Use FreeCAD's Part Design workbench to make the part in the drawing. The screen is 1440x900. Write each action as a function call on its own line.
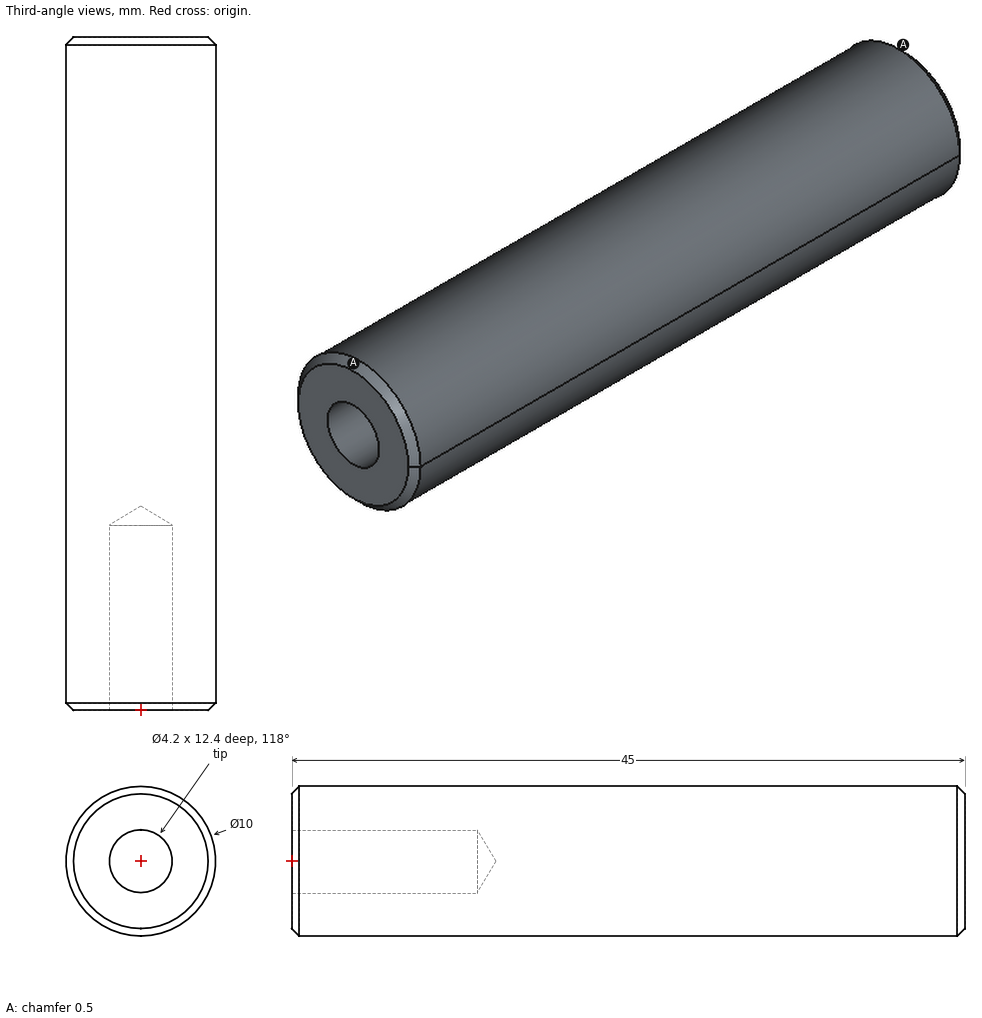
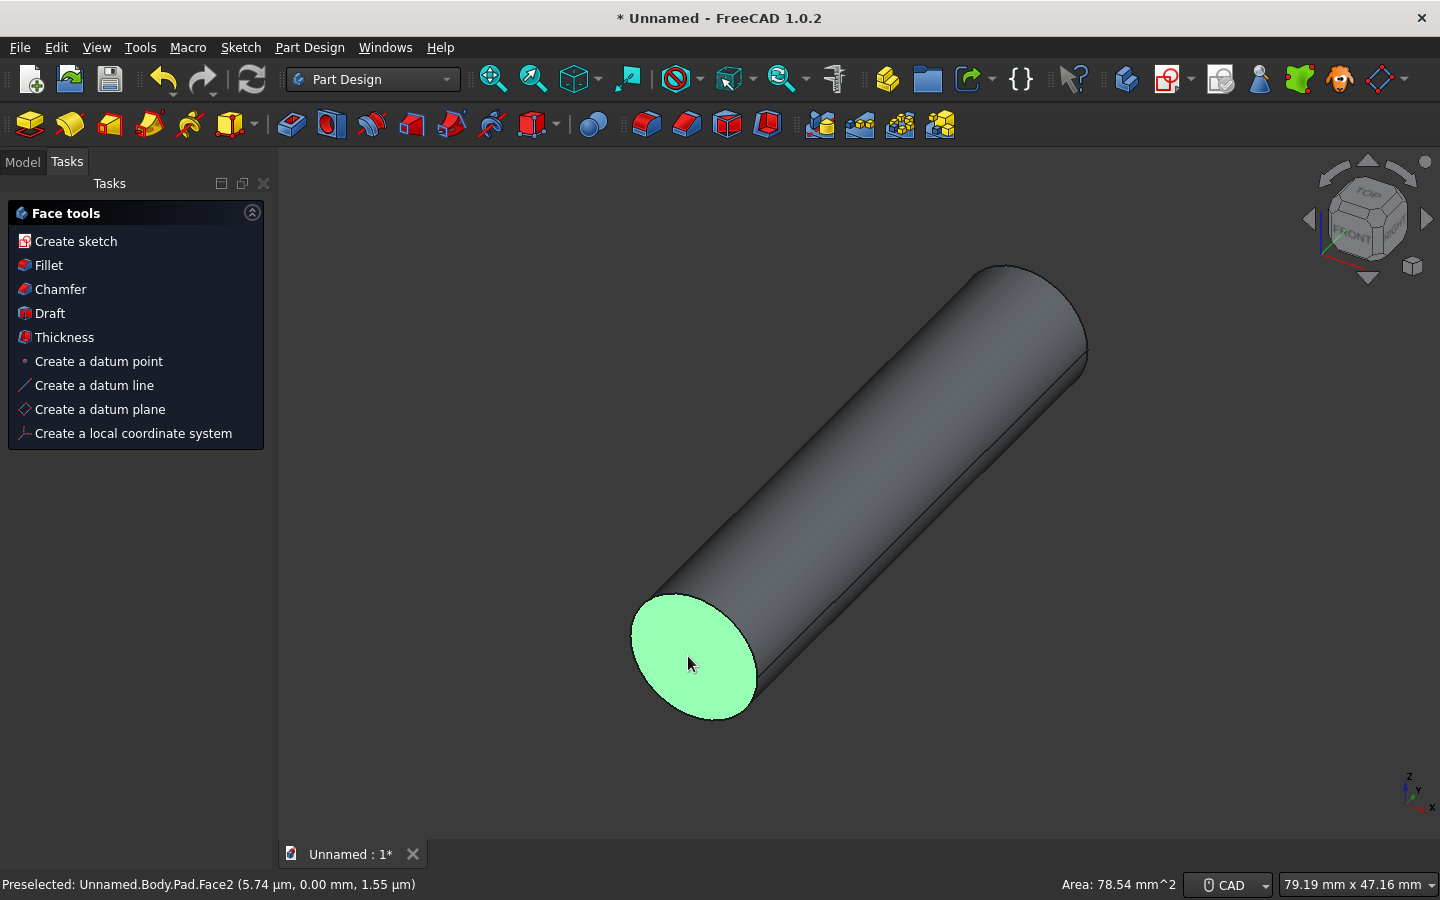
click(1168, 80)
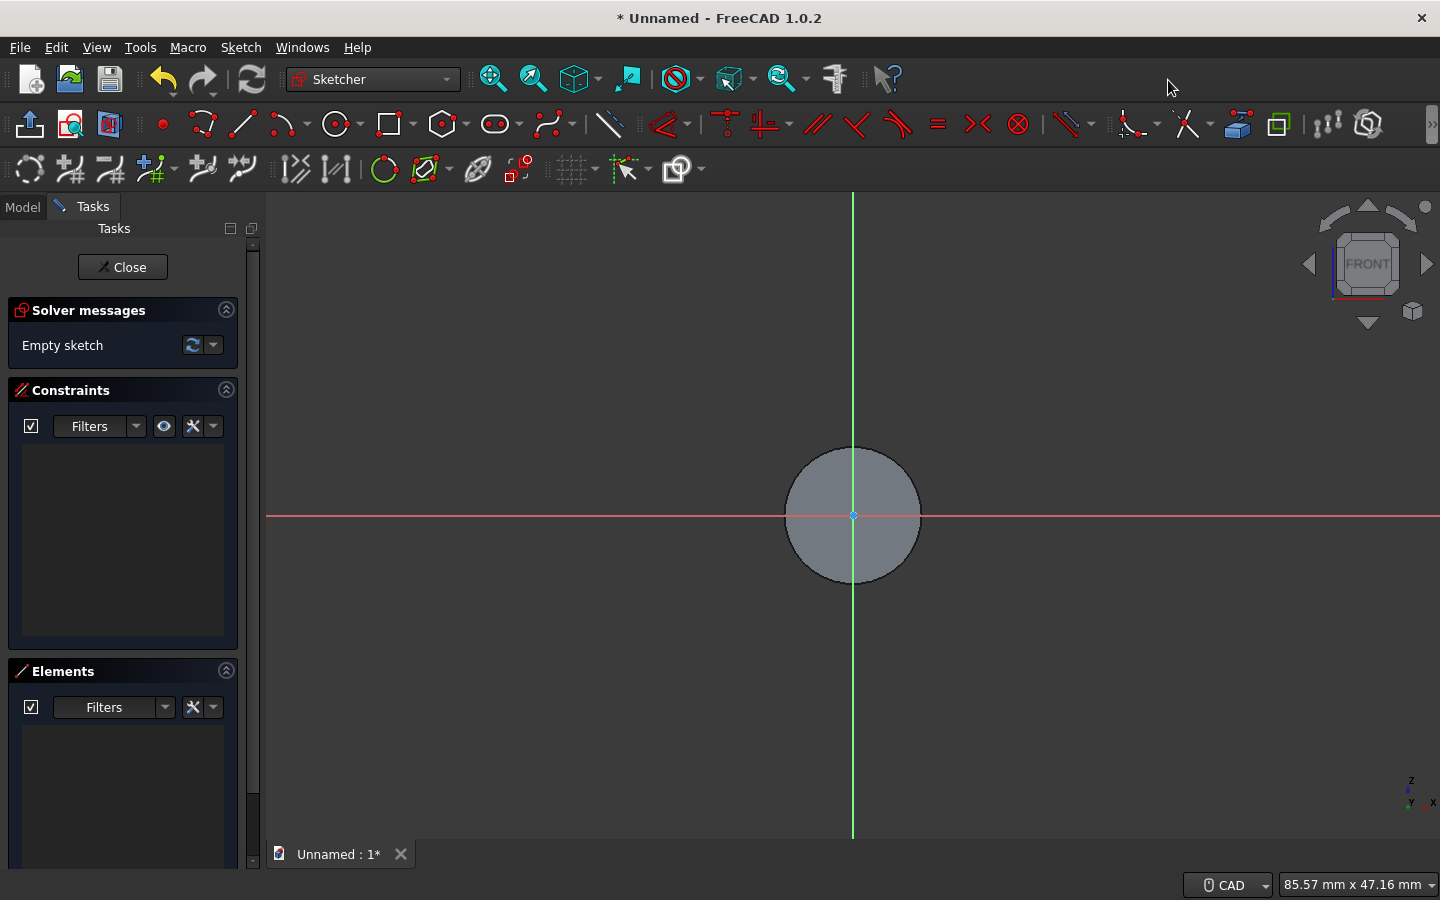
scroll(864, 516, up, 10)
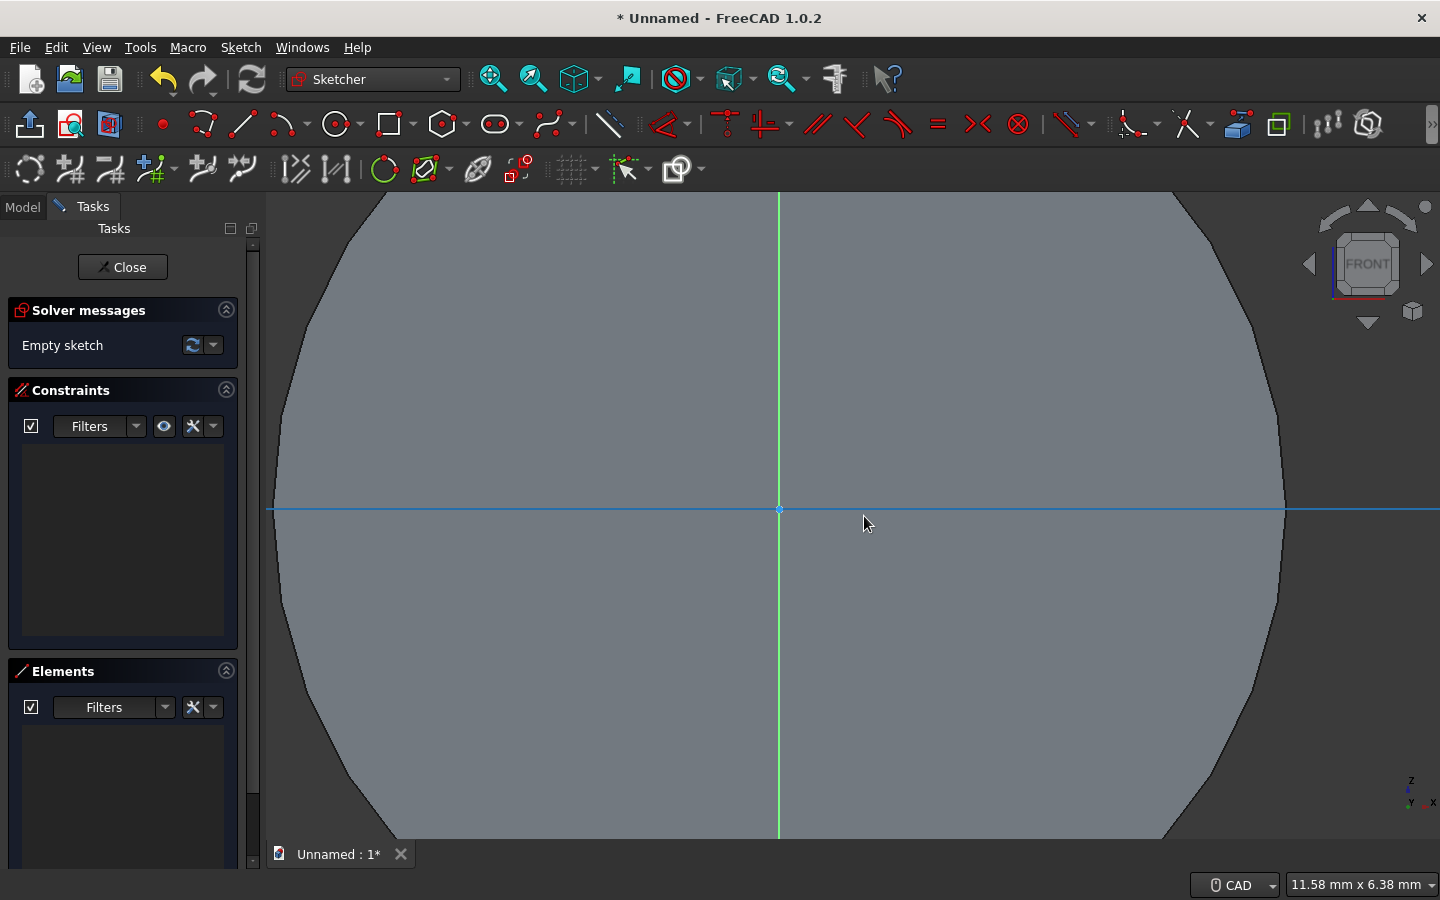
click(336, 124)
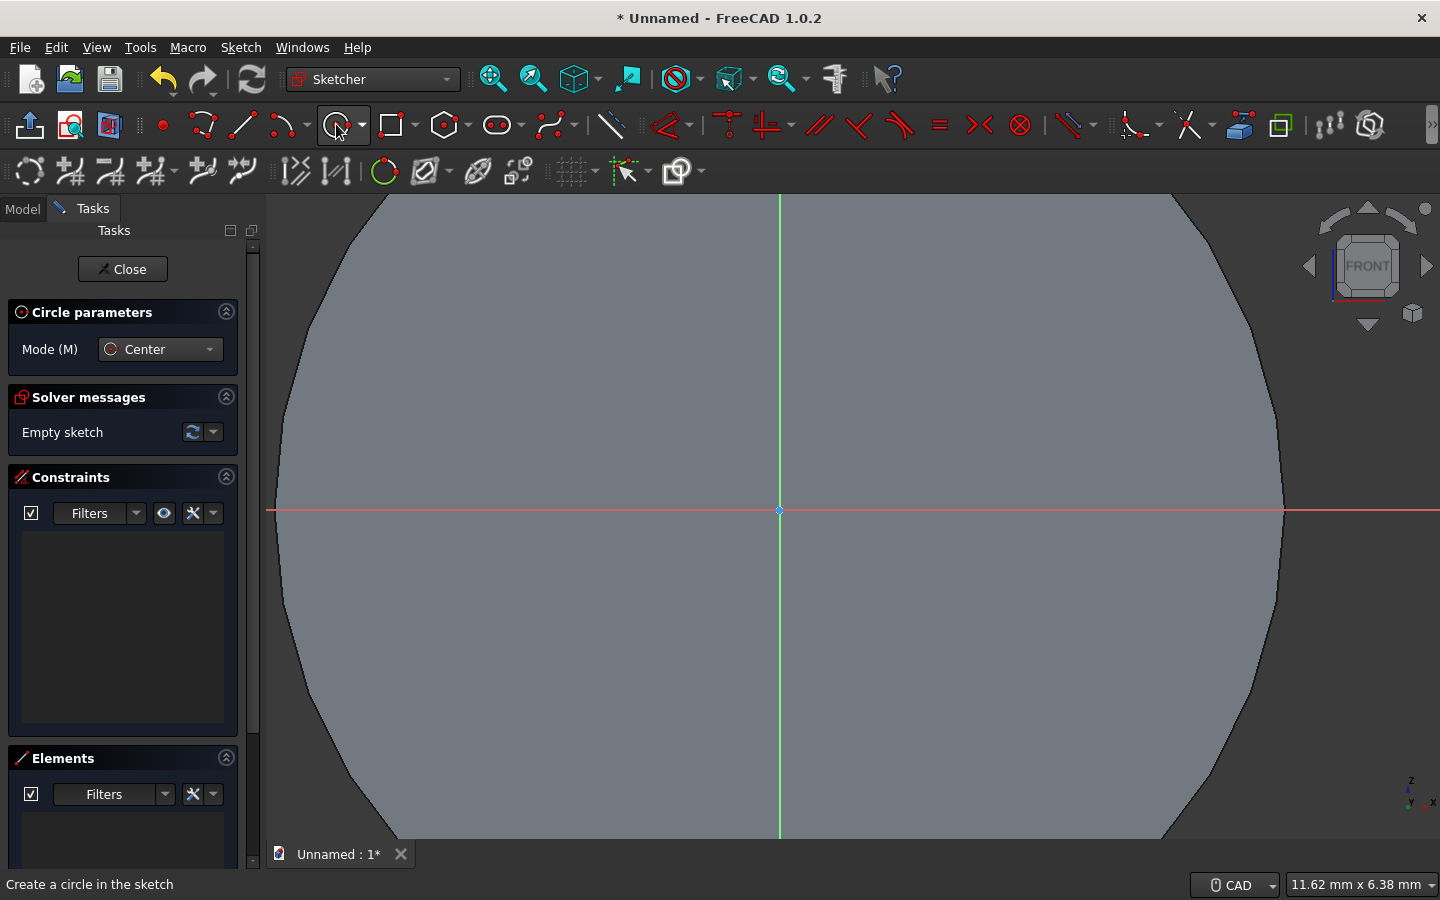
click(780, 510)
move(930, 360)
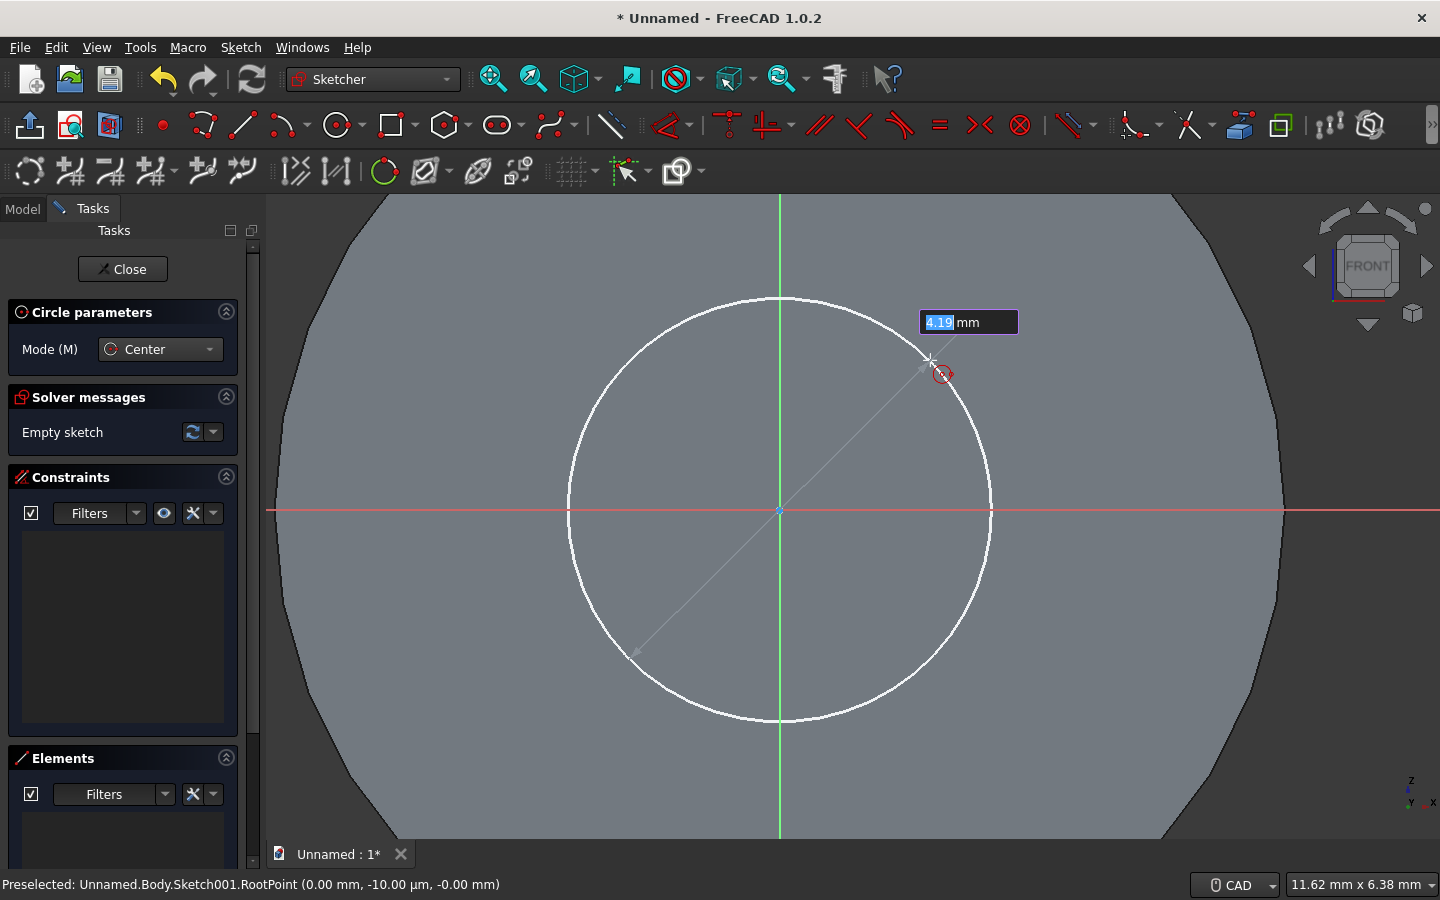
text(4.2)
key(Return)
key(Escape)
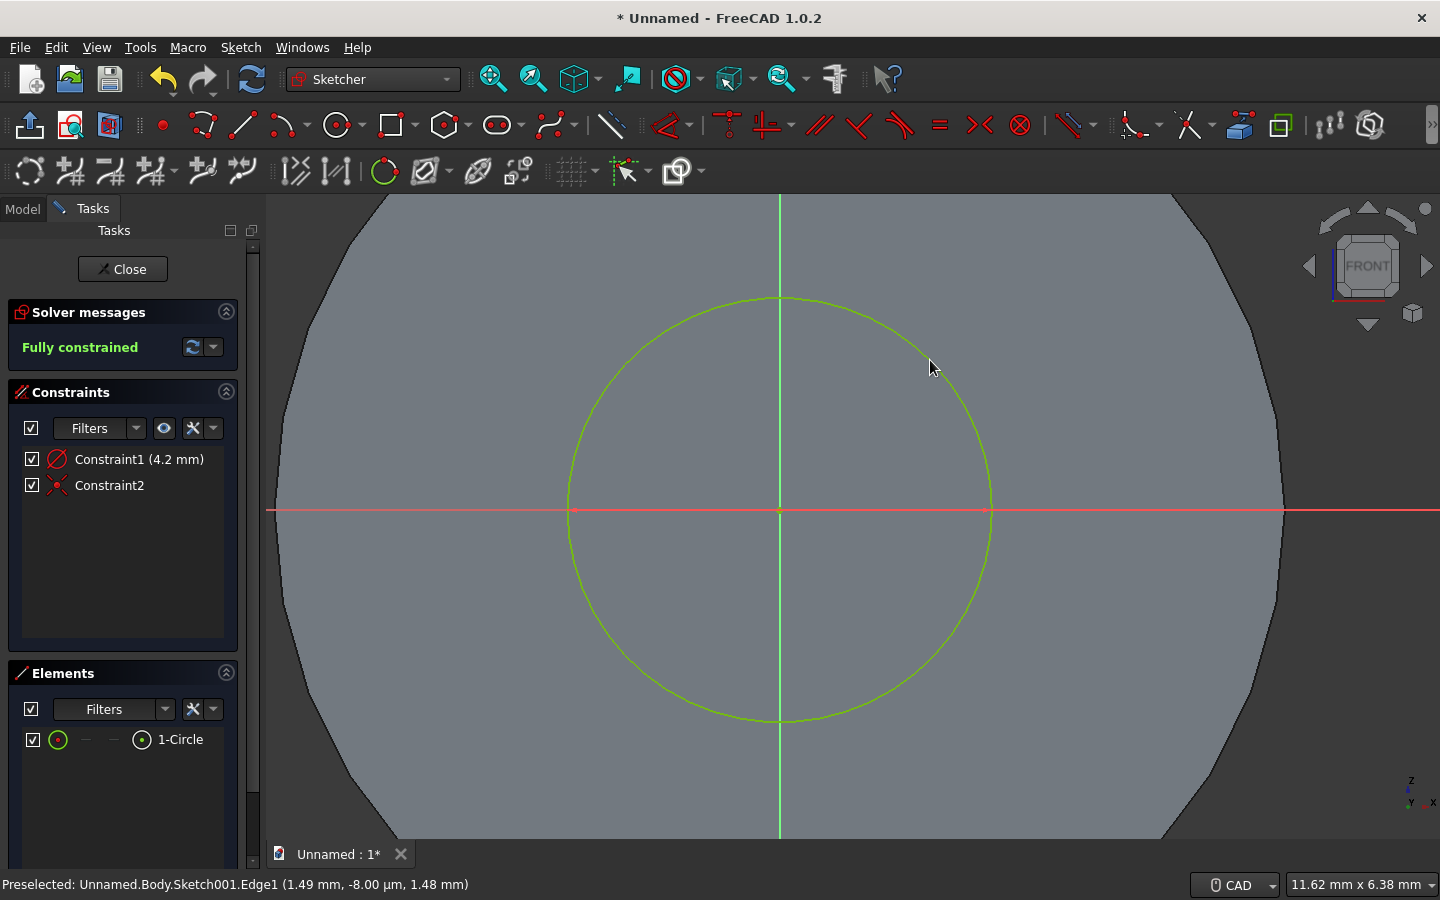
click(123, 269)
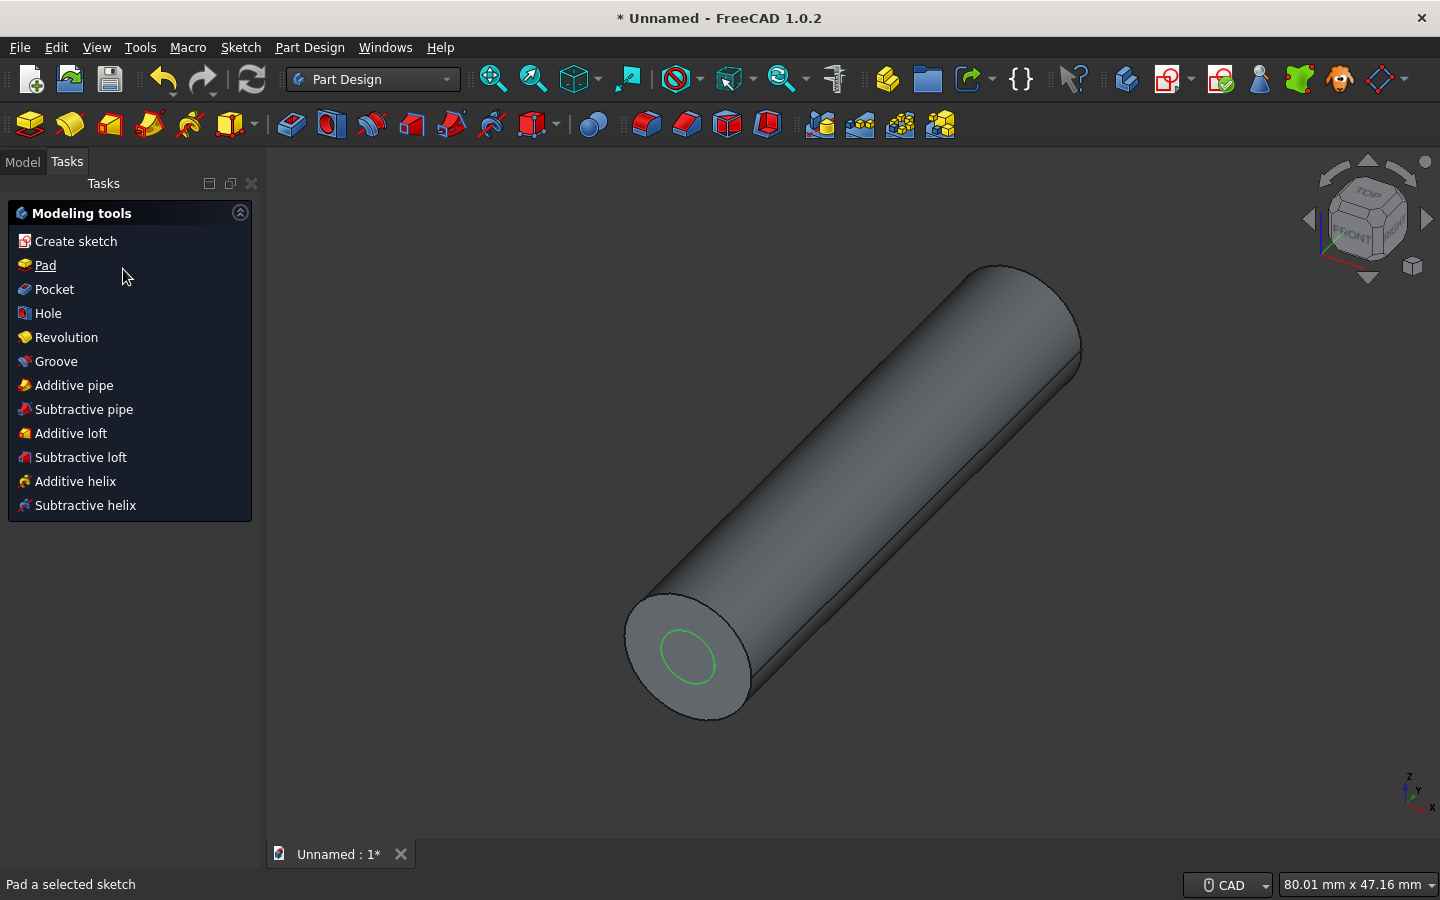
click(332, 124)